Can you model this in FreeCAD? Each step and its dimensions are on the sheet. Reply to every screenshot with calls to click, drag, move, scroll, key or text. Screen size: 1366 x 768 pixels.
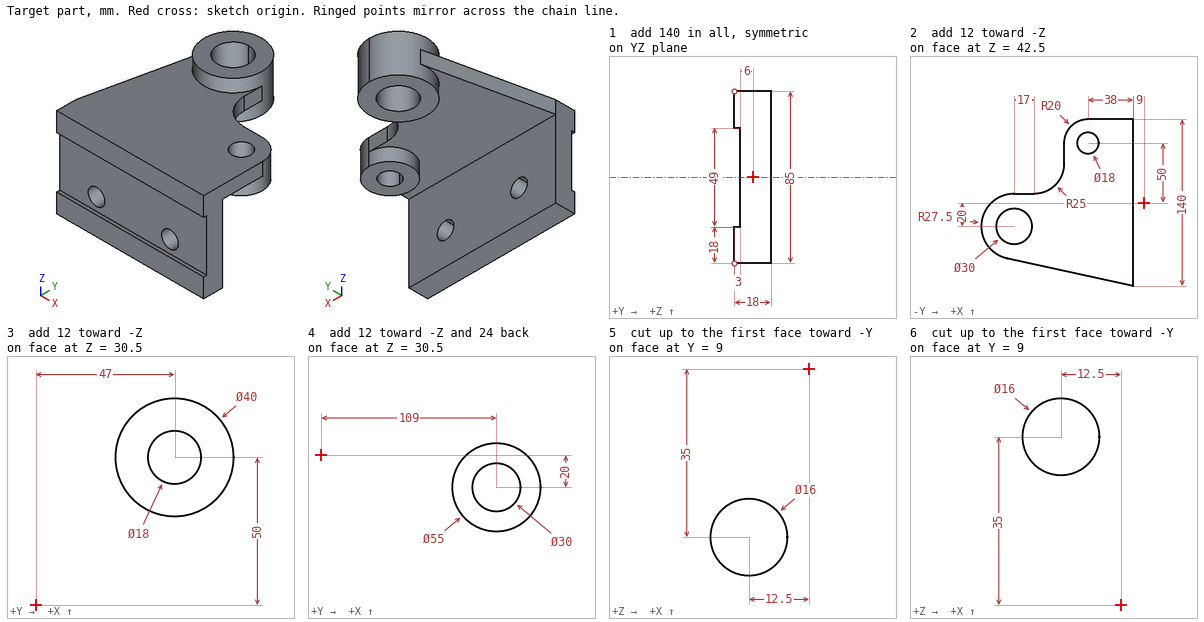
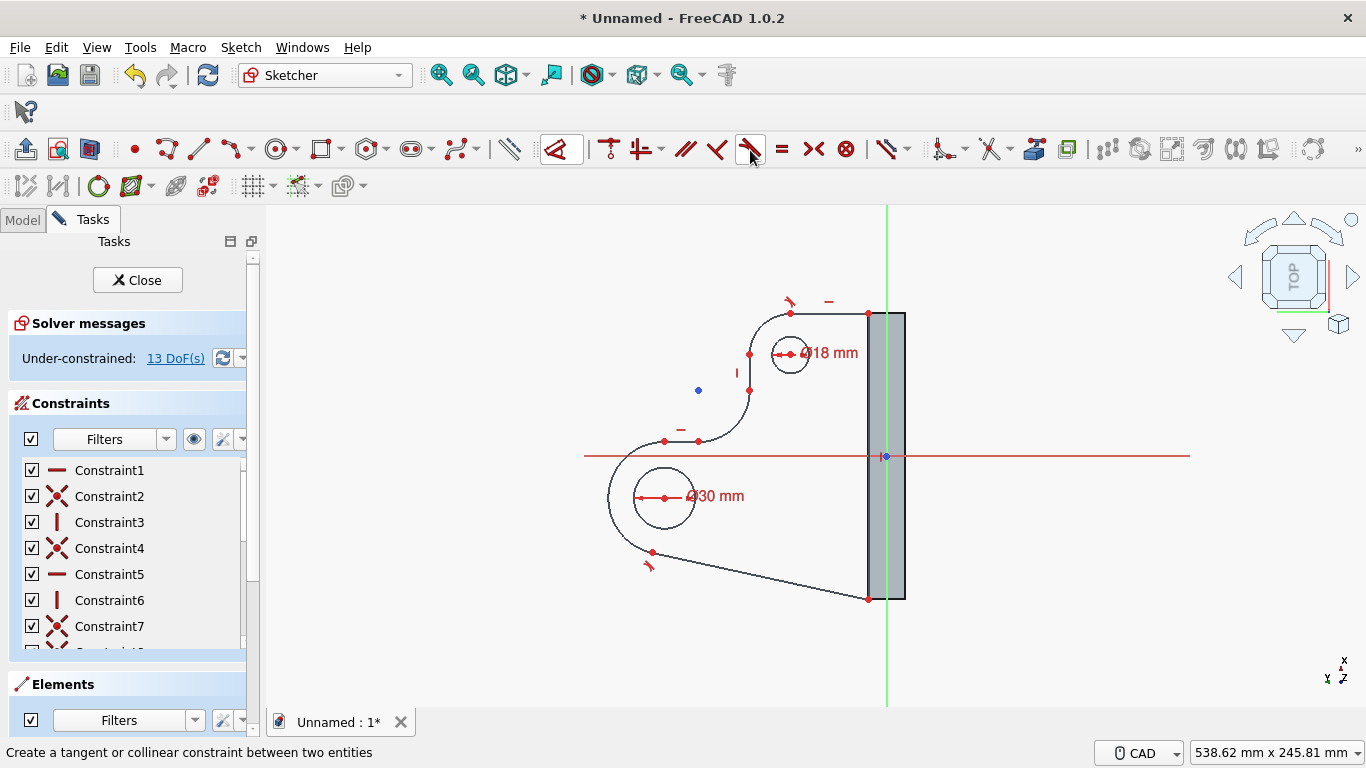
scroll(675, 442, up, 2)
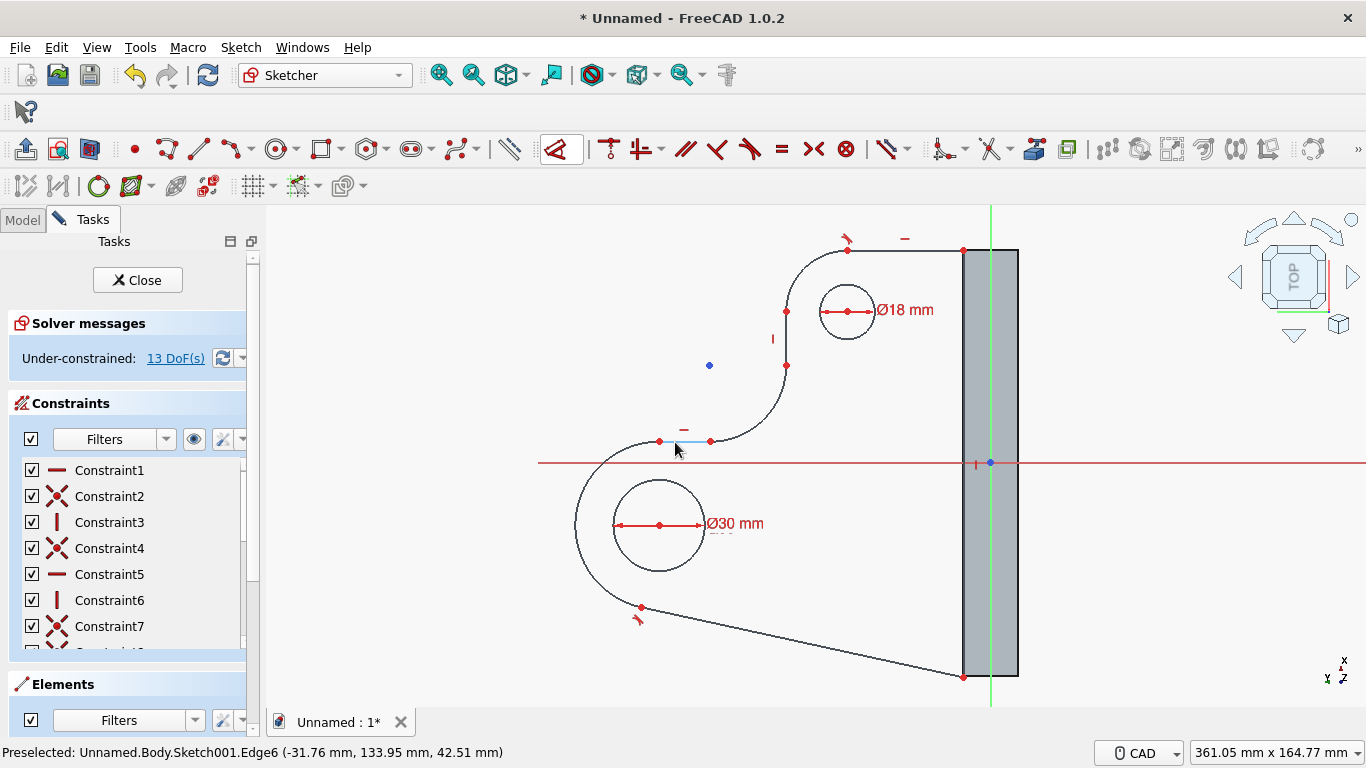
click(675, 442)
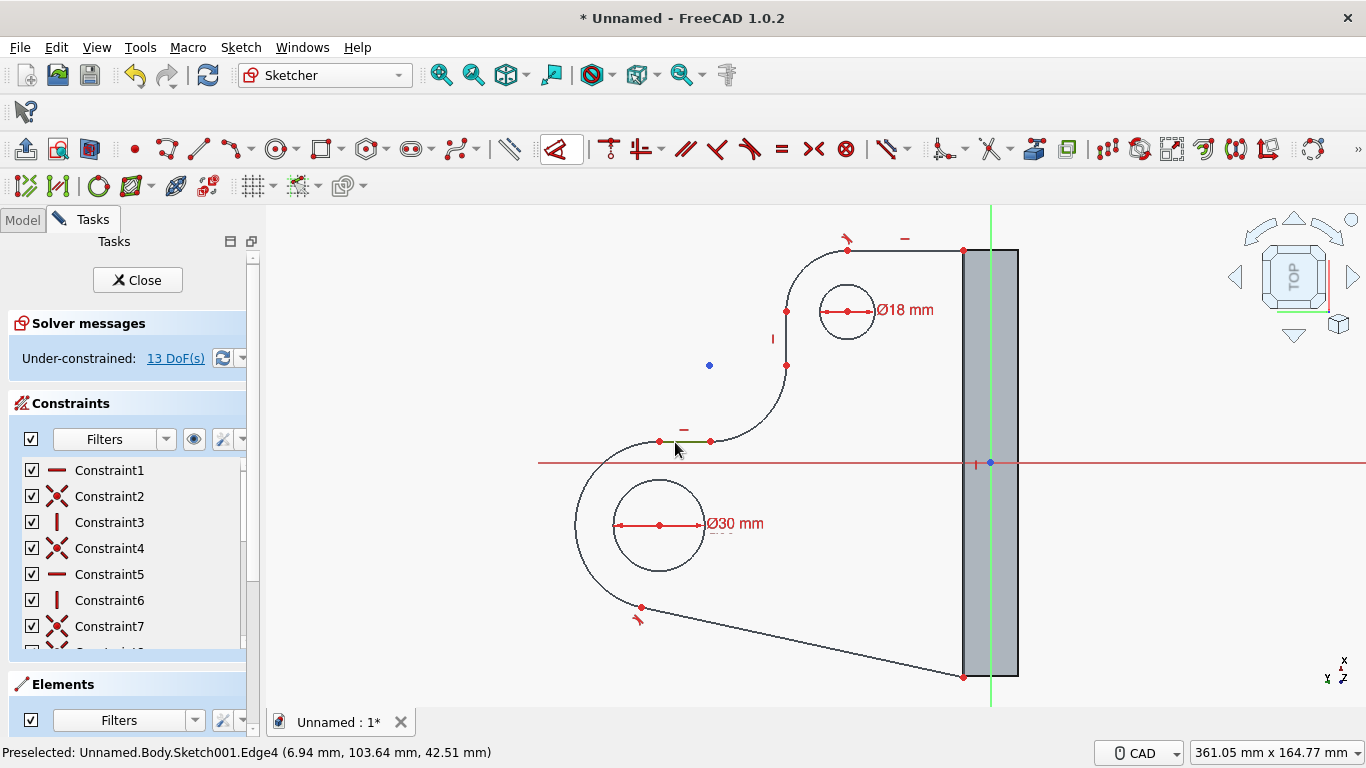
click(585, 564)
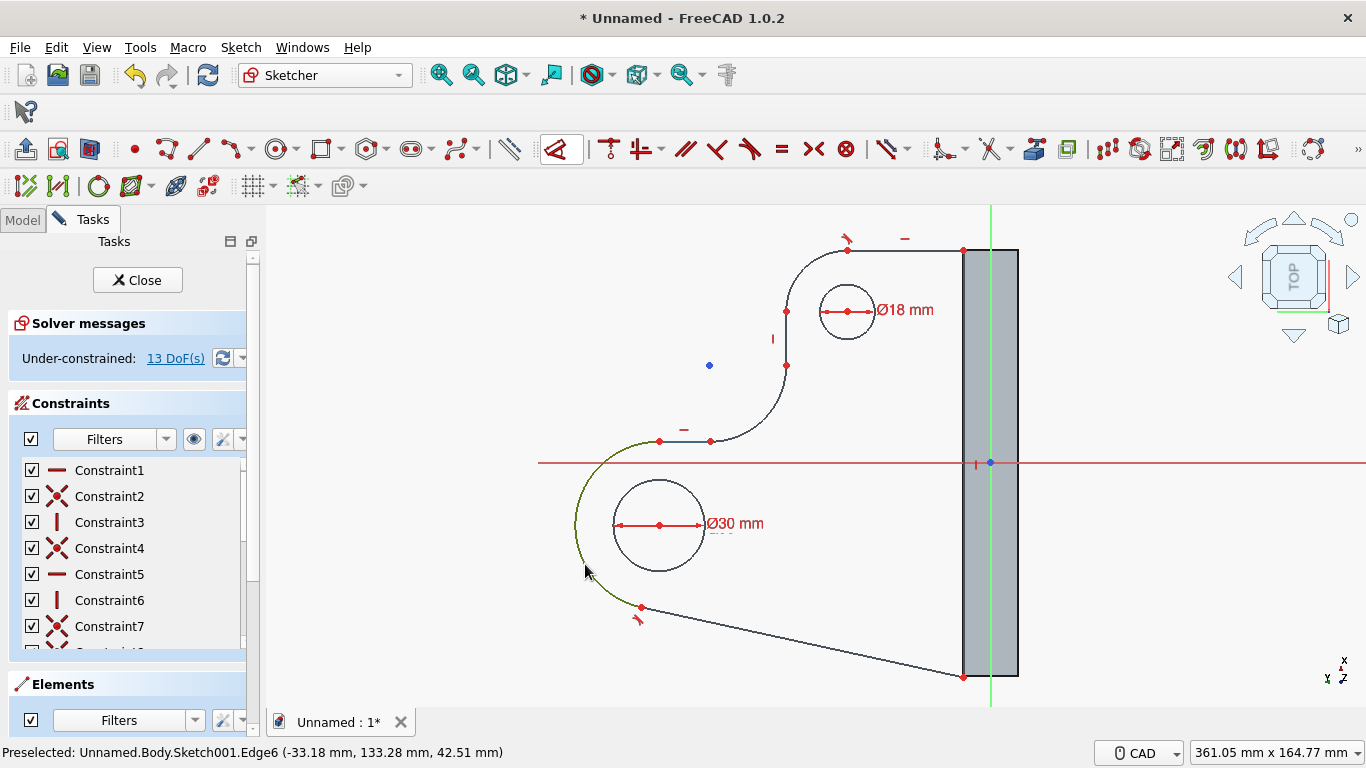
key(t)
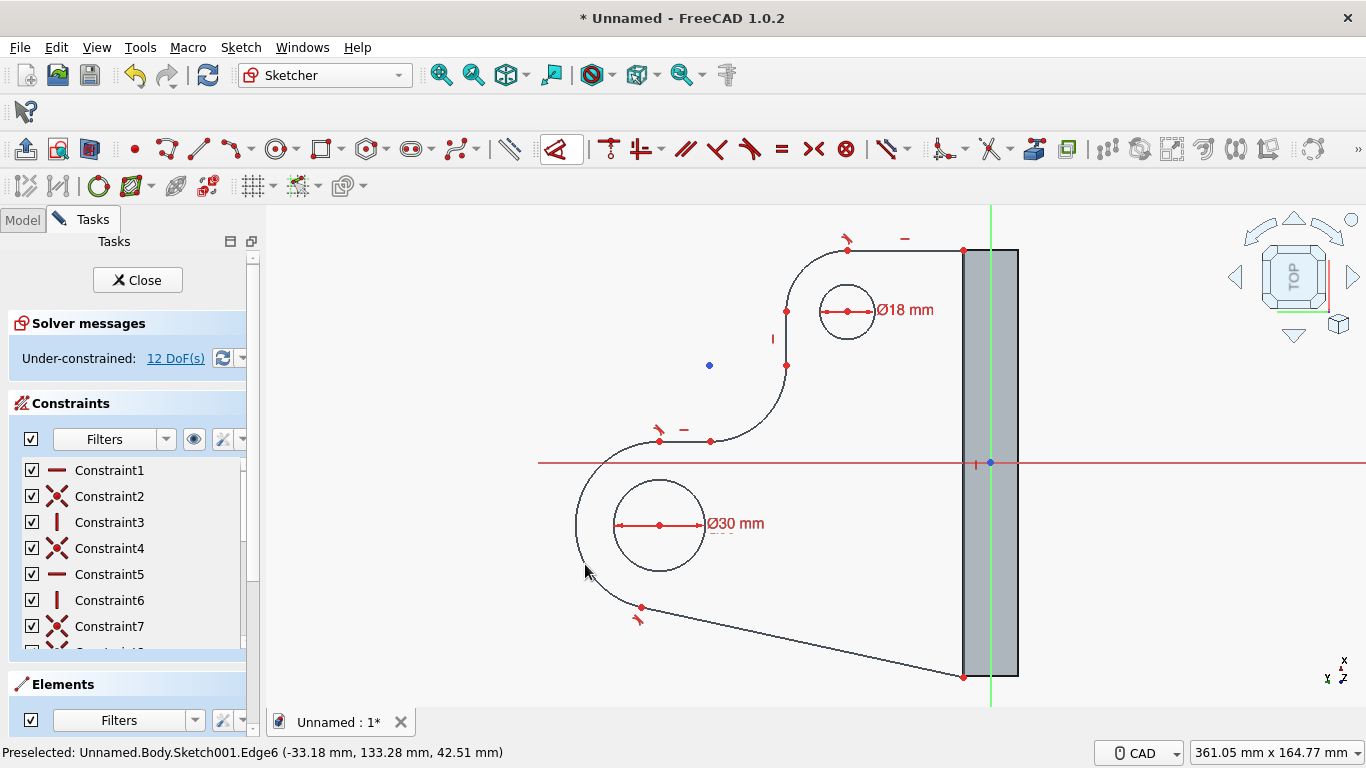
click(675, 442)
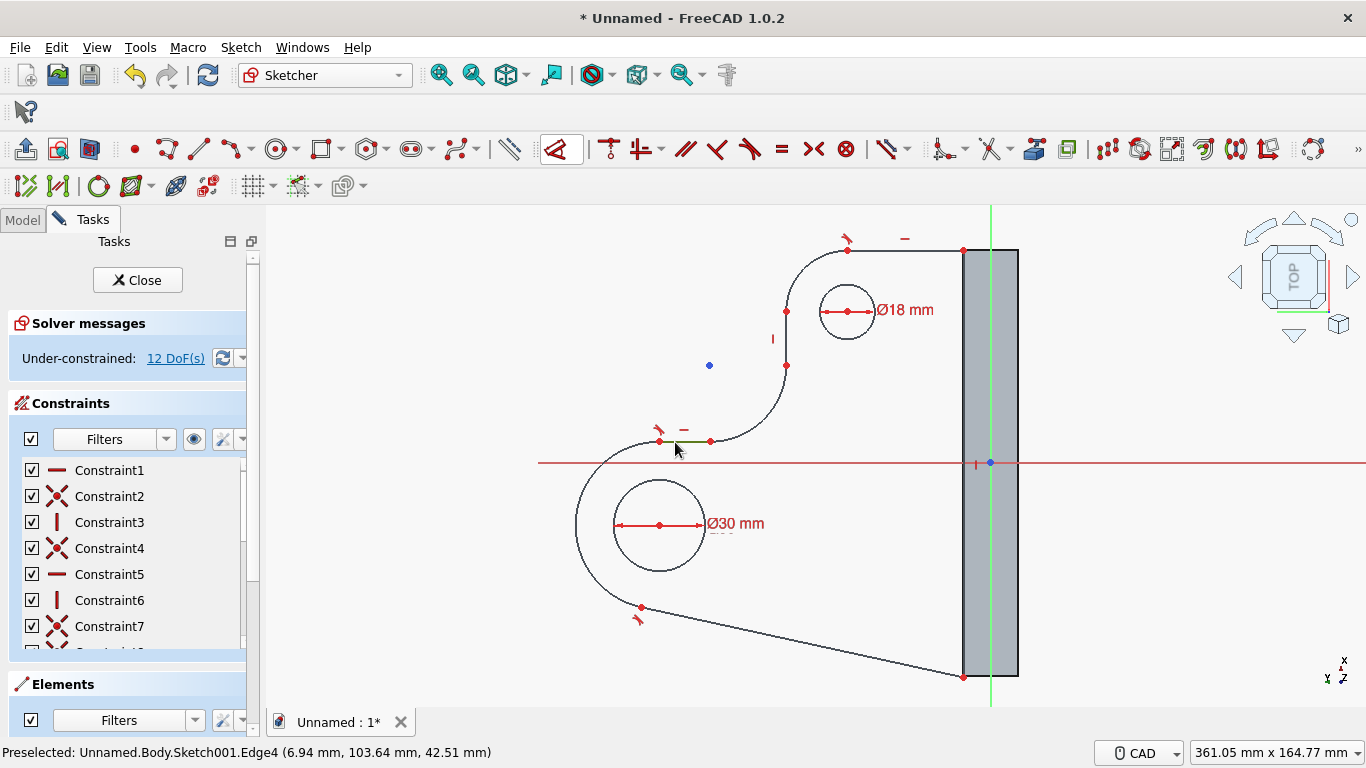
click(745, 433)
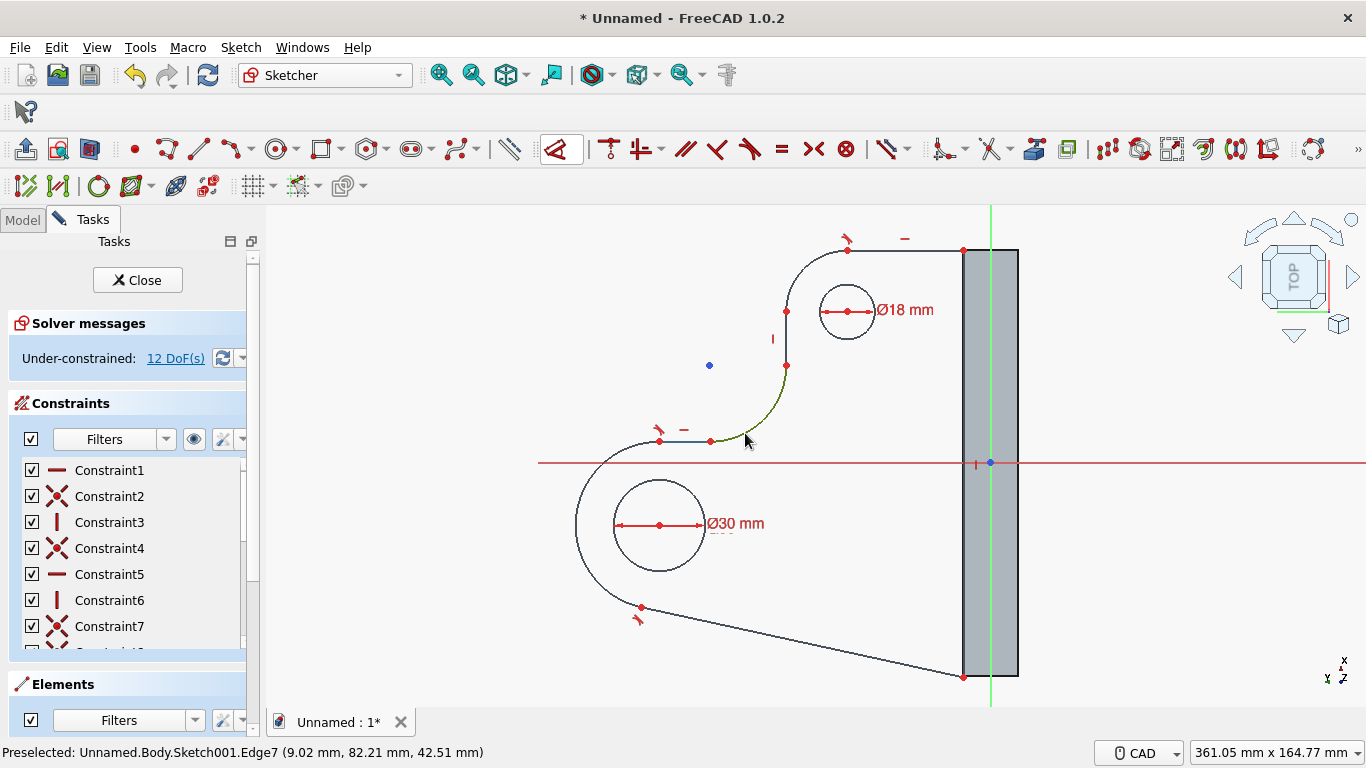
click(750, 150)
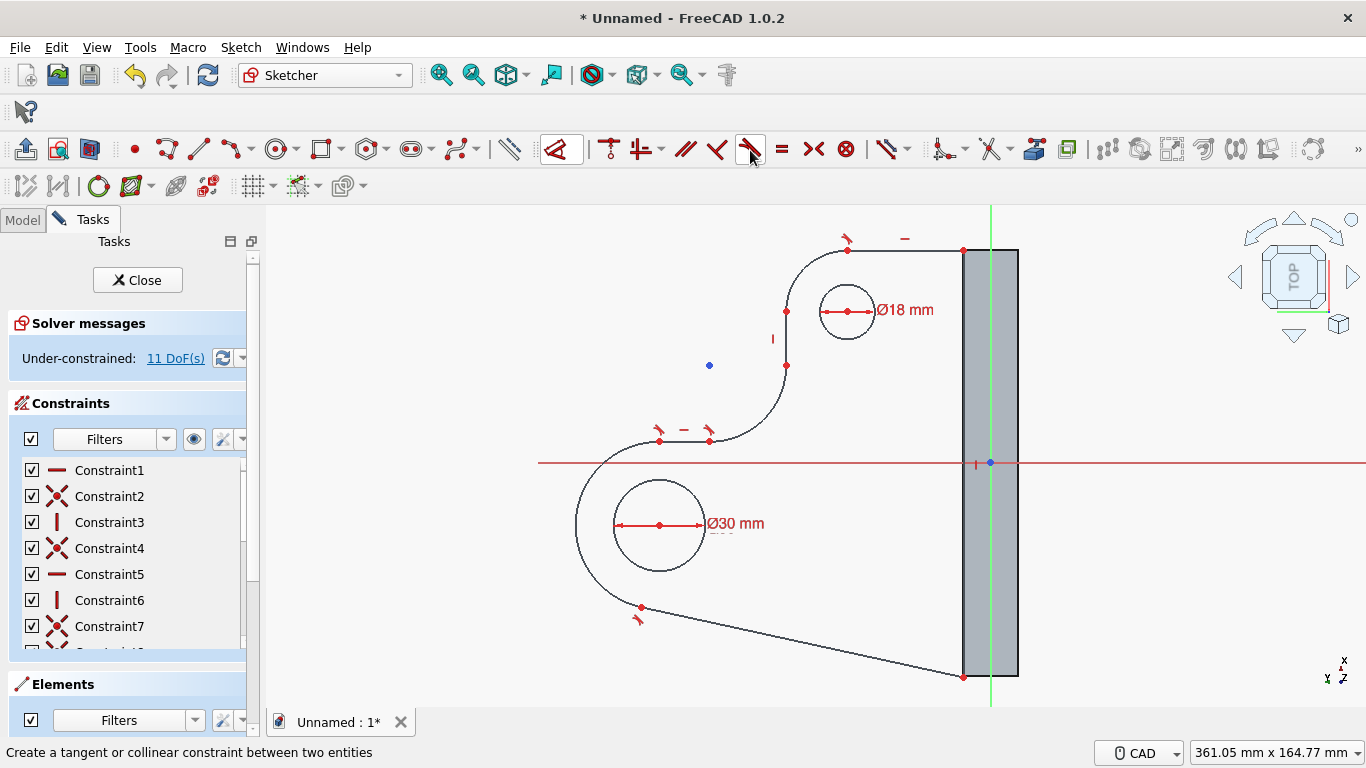
click(786, 350)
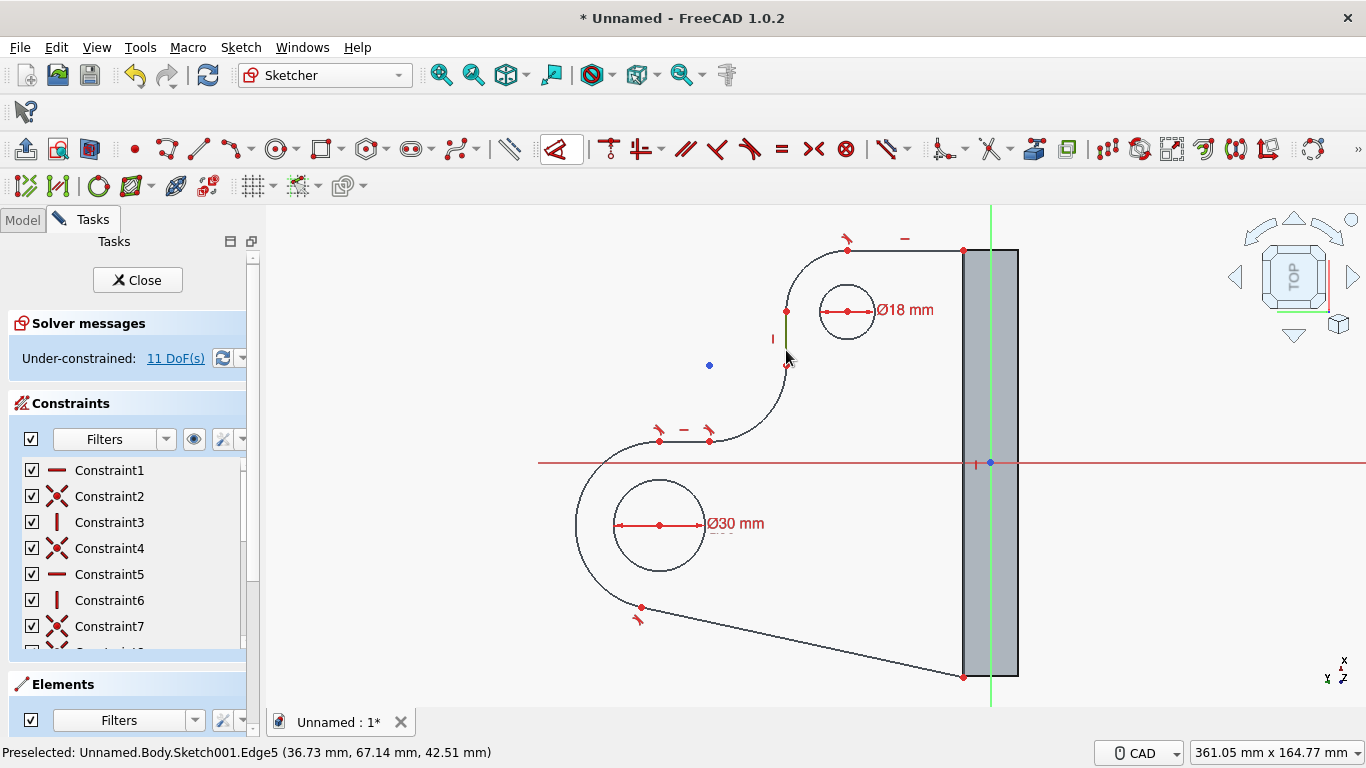
click(744, 433)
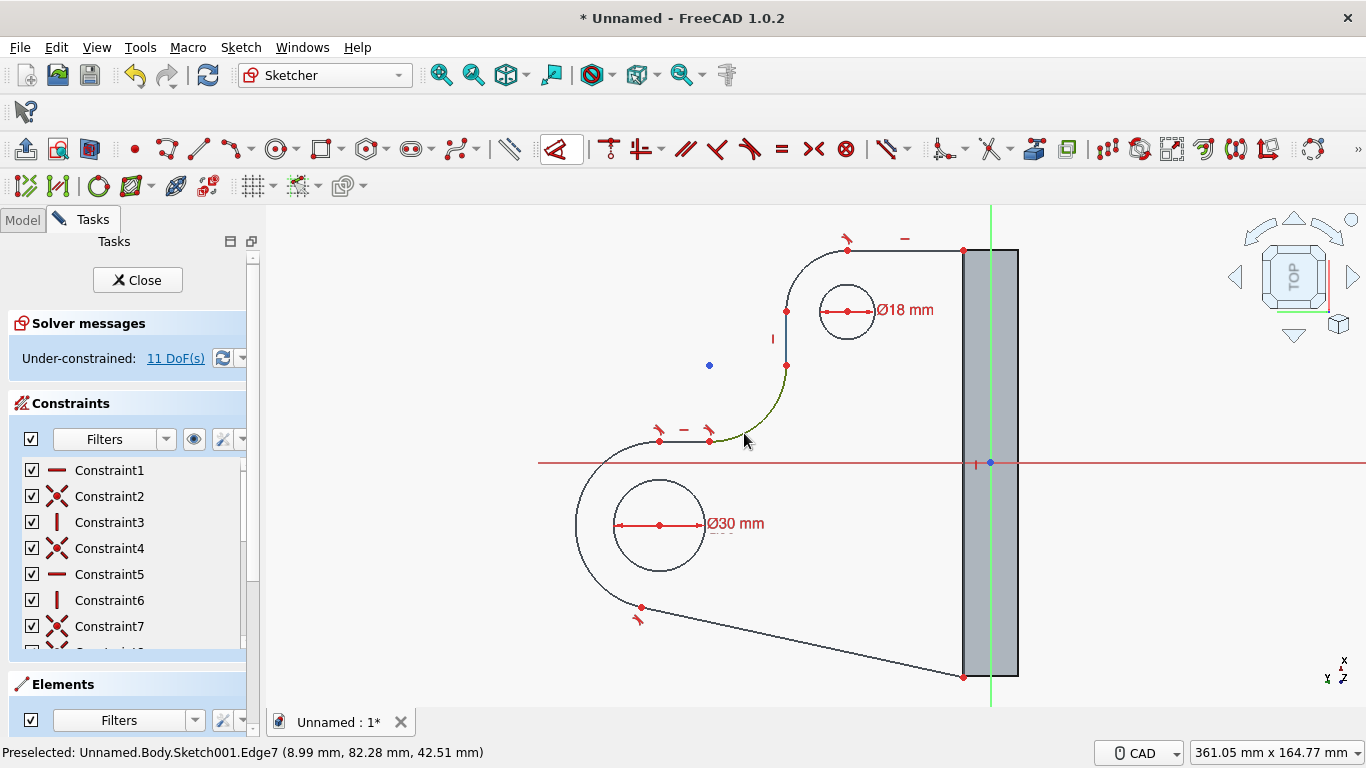
key(t)